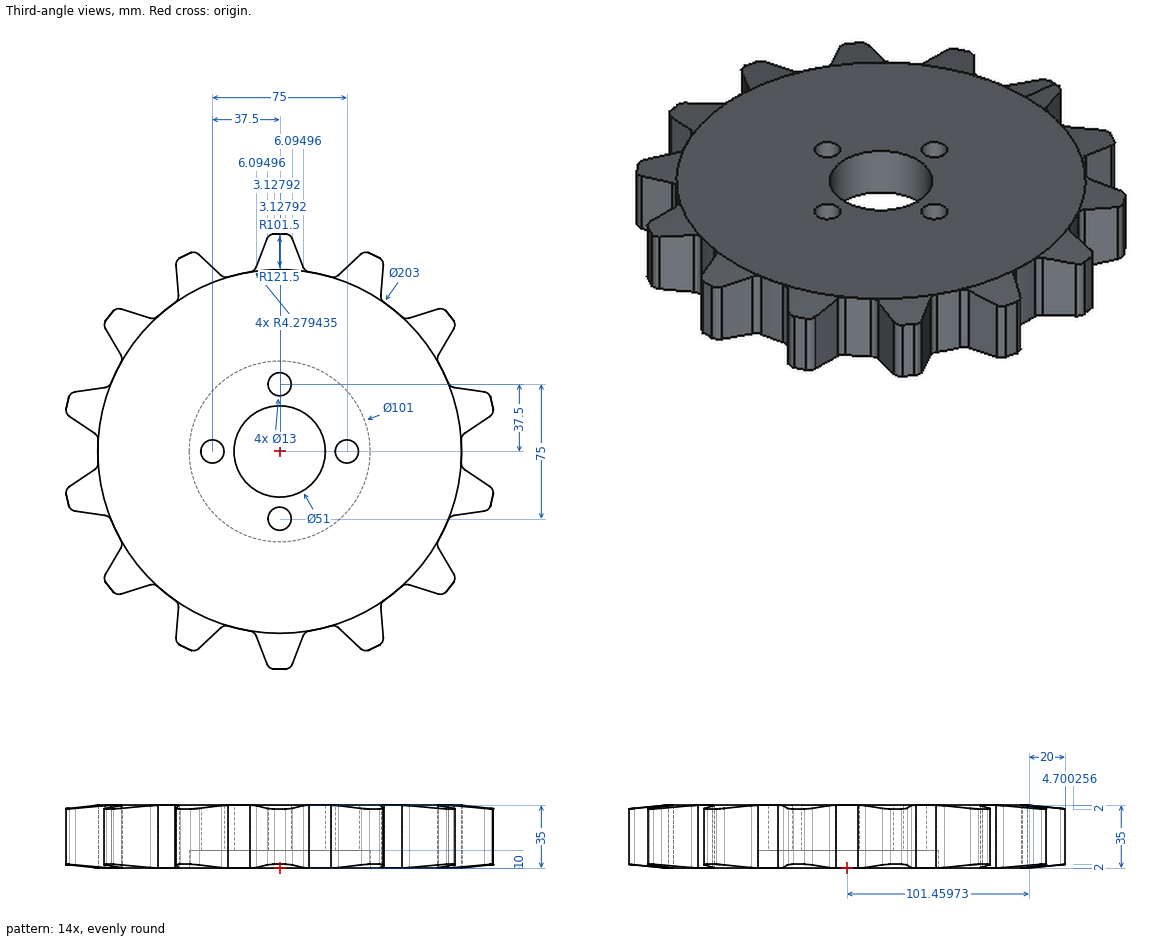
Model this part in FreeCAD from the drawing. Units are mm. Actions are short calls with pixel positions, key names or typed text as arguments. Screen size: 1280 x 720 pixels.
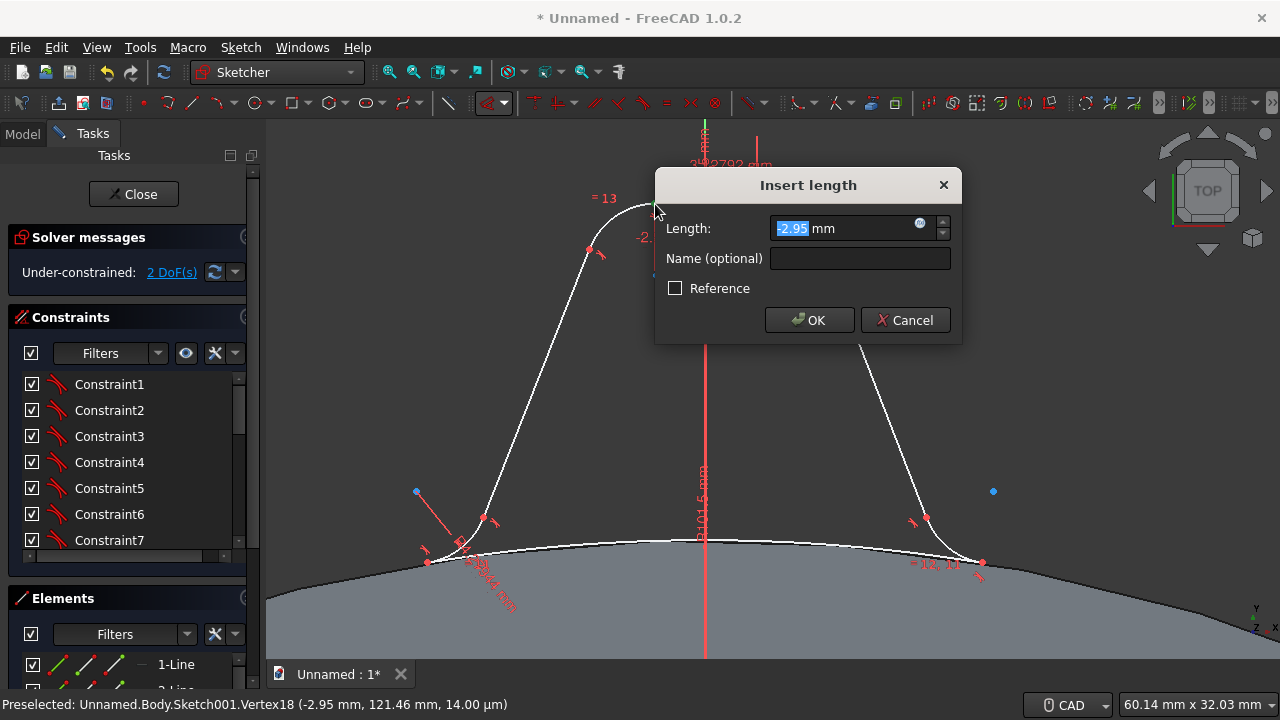
text(-3.12792)
key(Return)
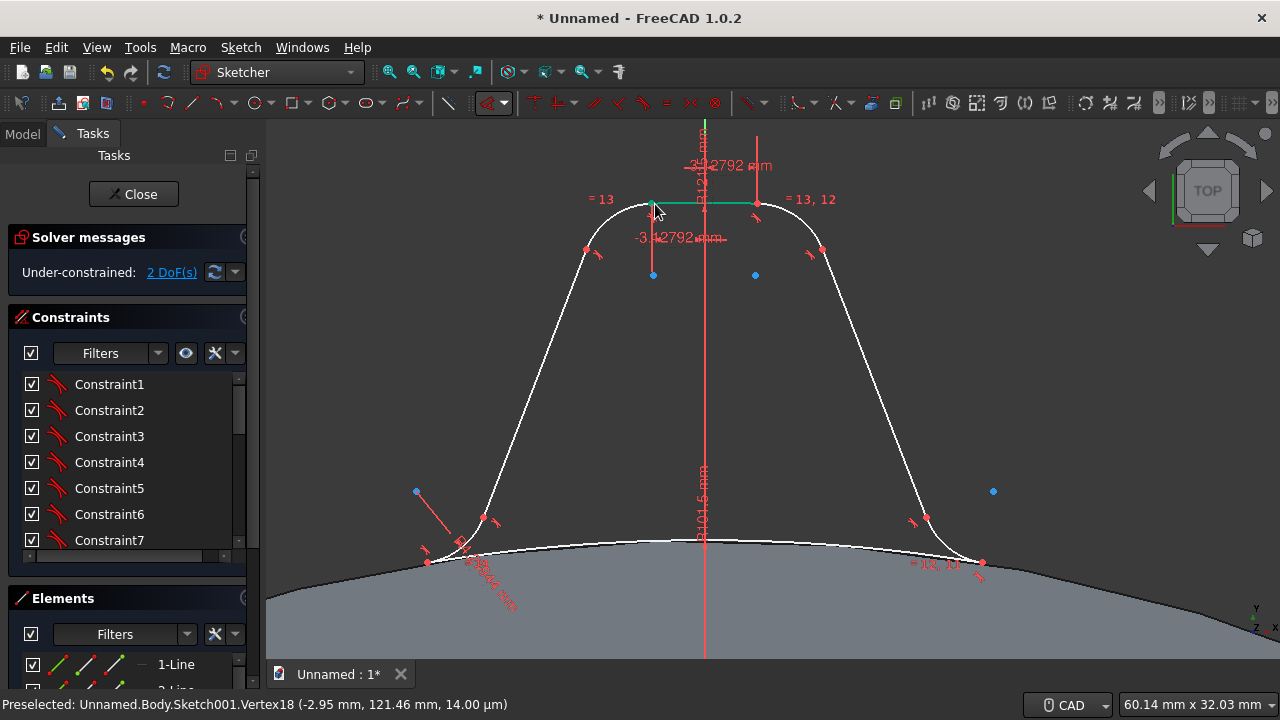
click(556, 330)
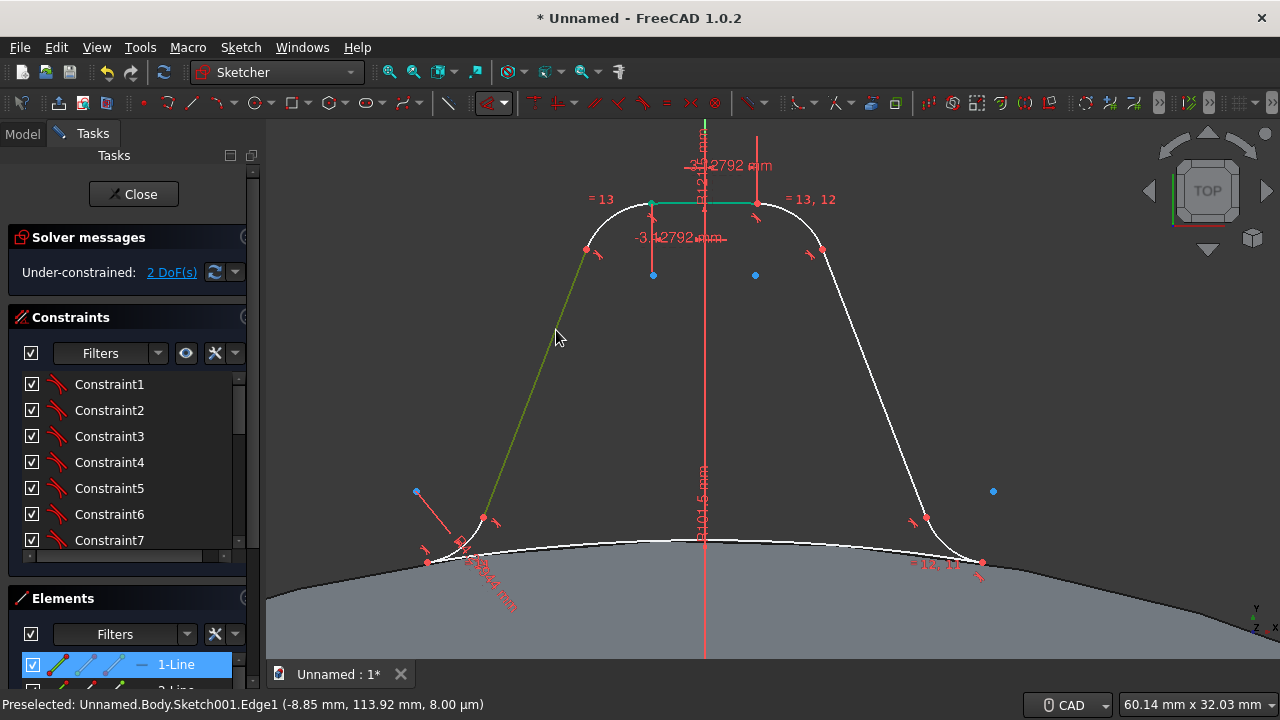
key(l)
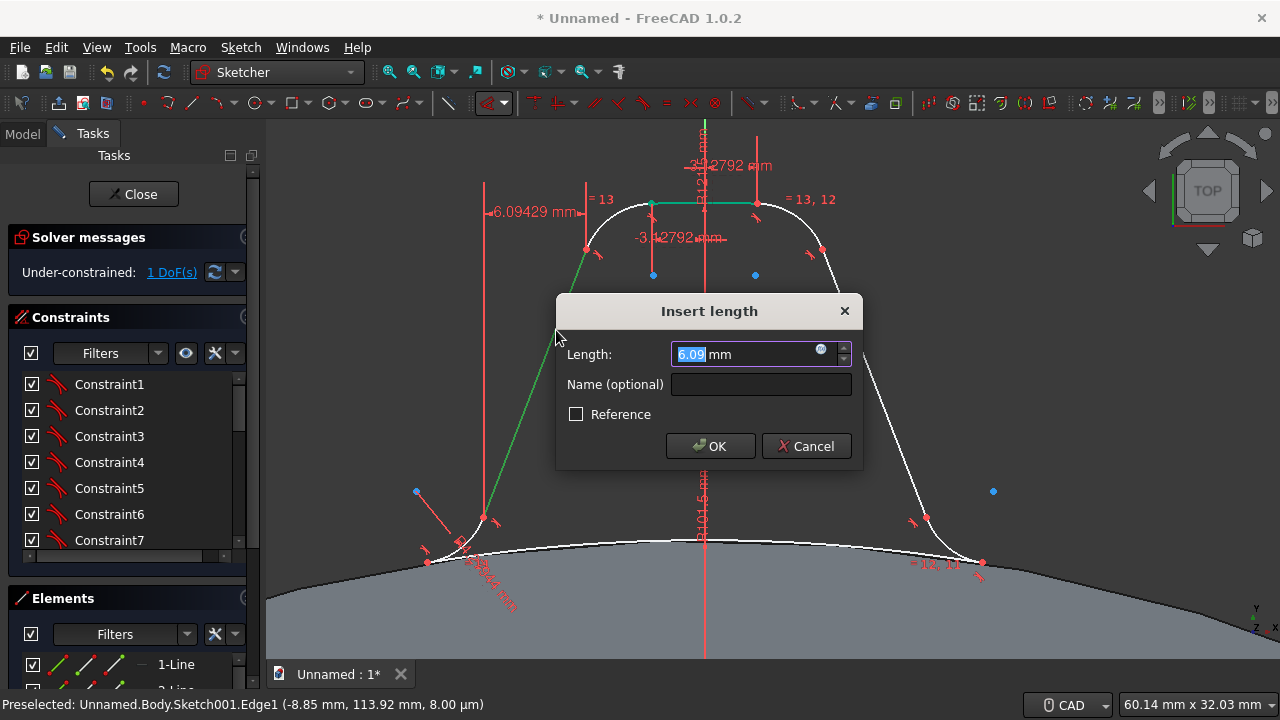
text(6.09496)
key(Return)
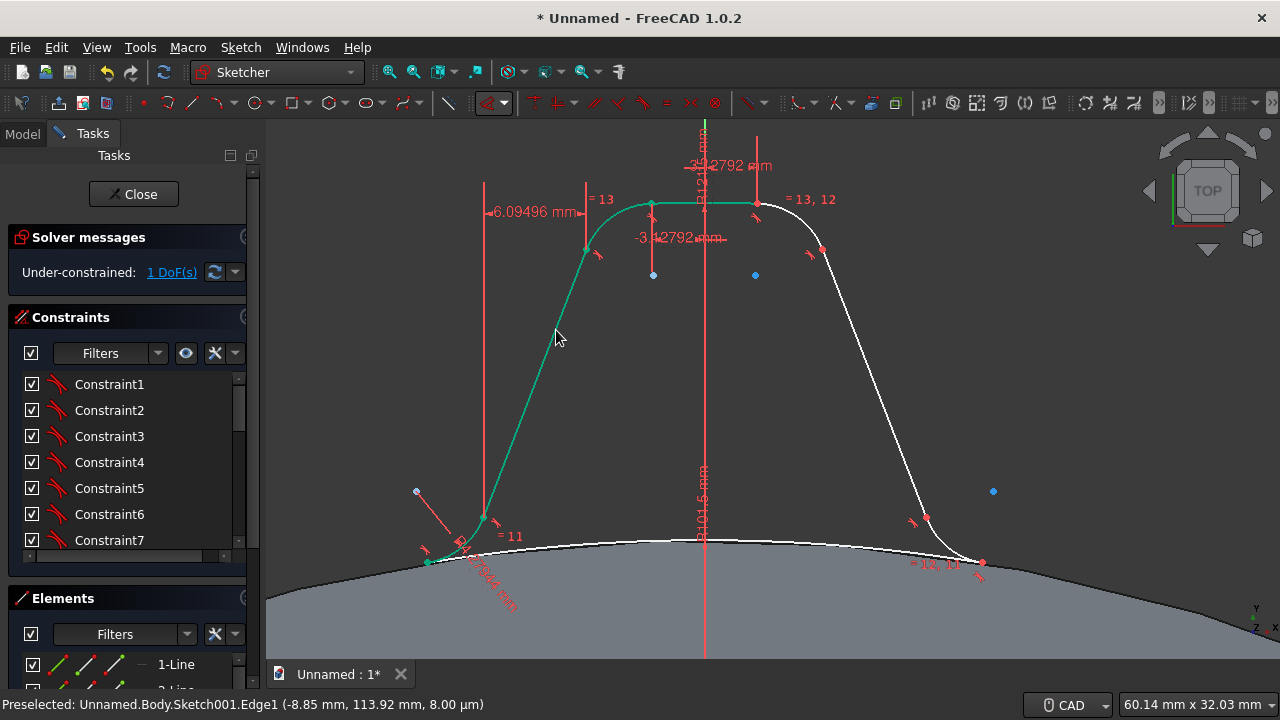
click(895, 437)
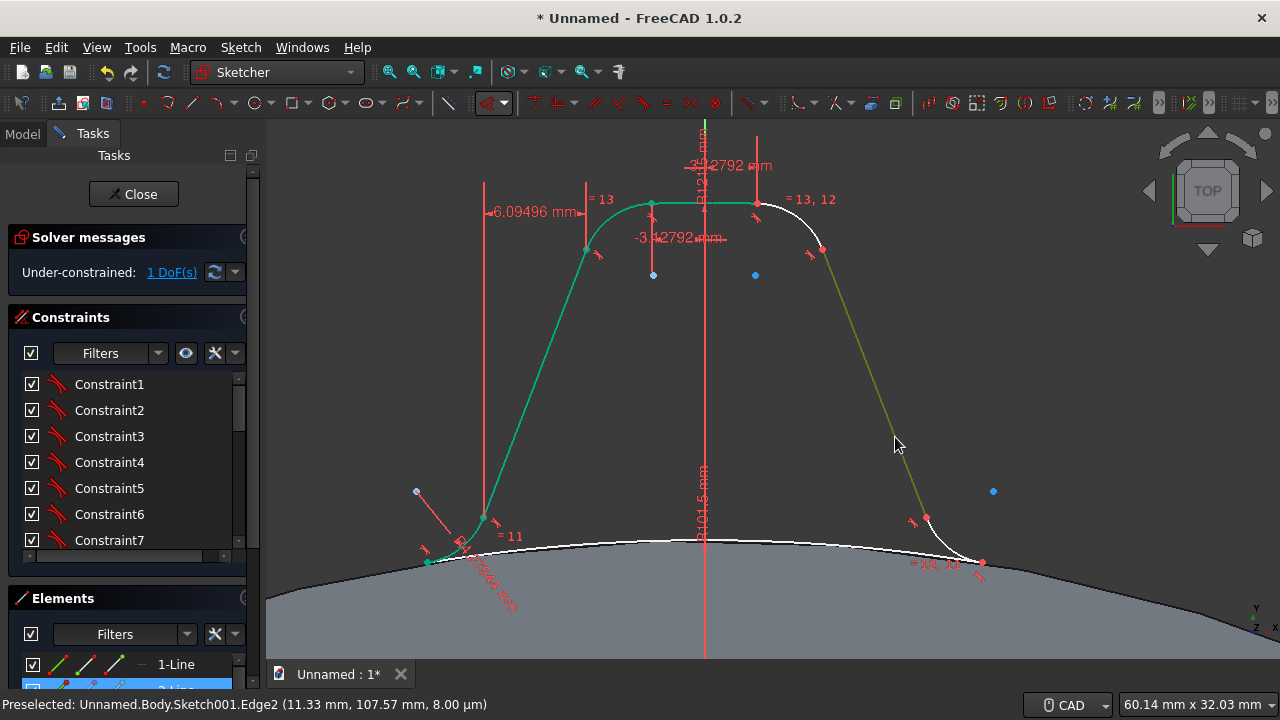
click(506, 104)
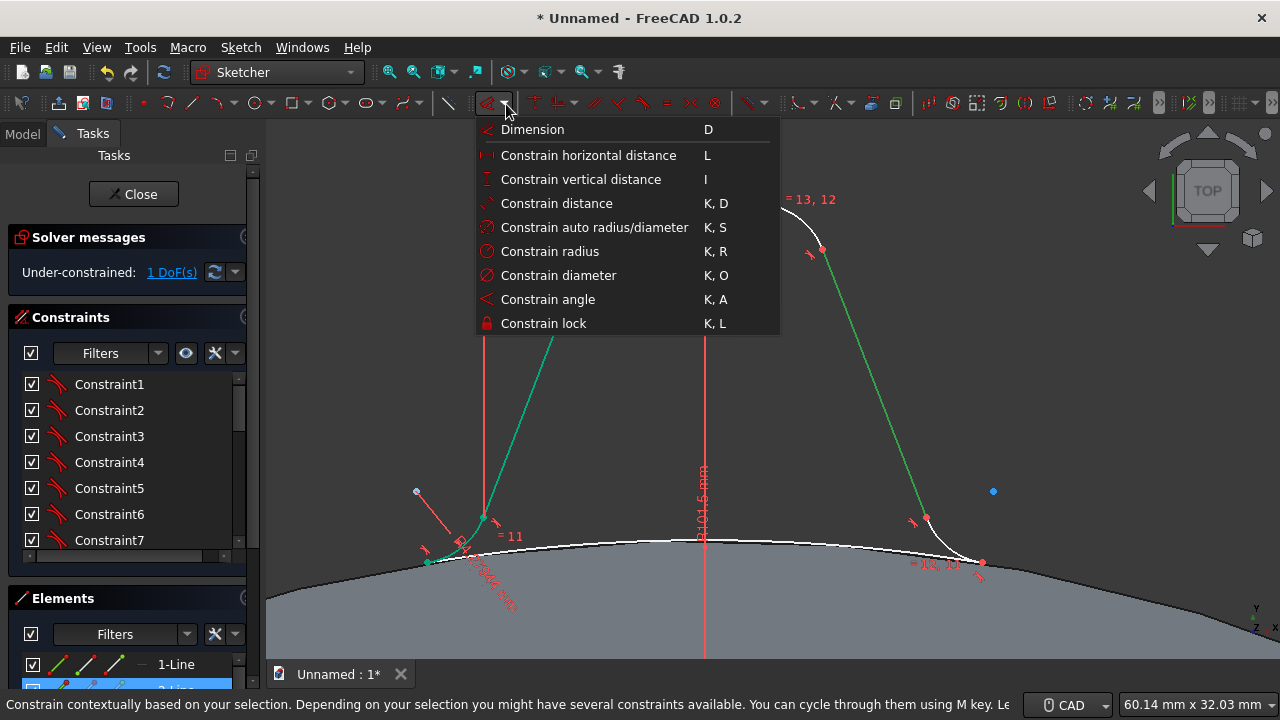
click(628, 155)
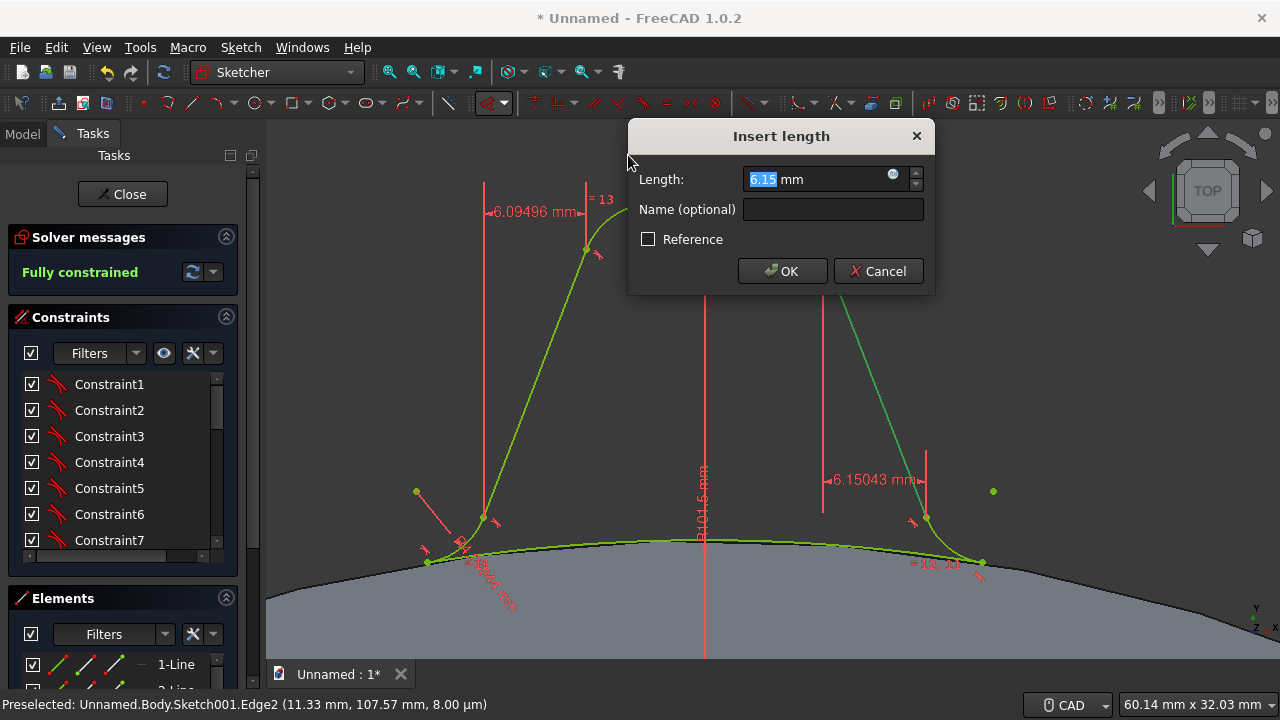
text(6.09496)
key(Return)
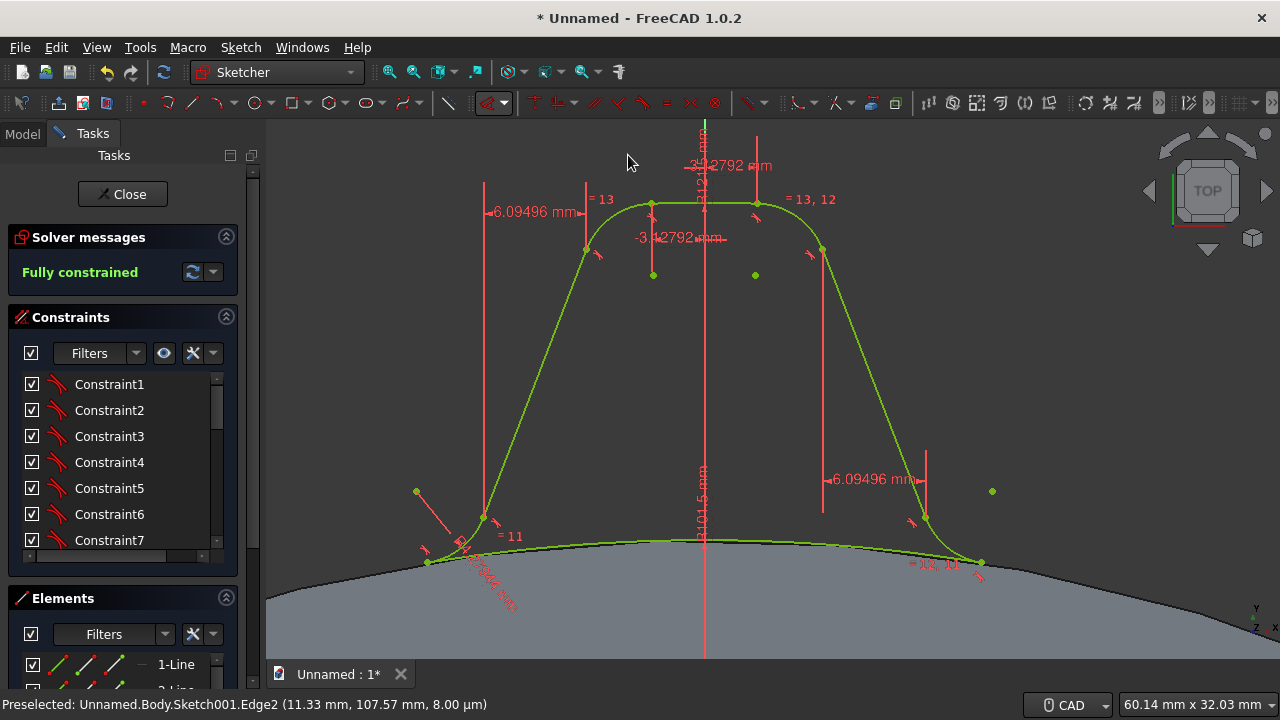
click(123, 194)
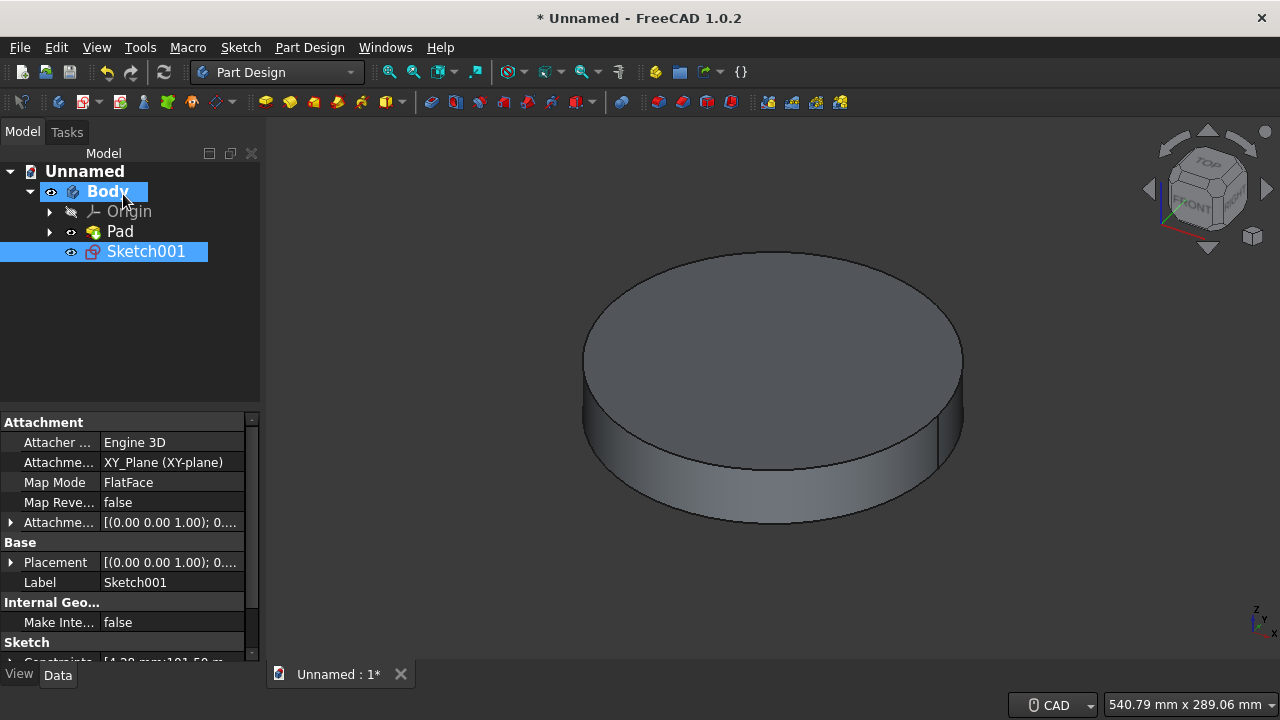
click(266, 102)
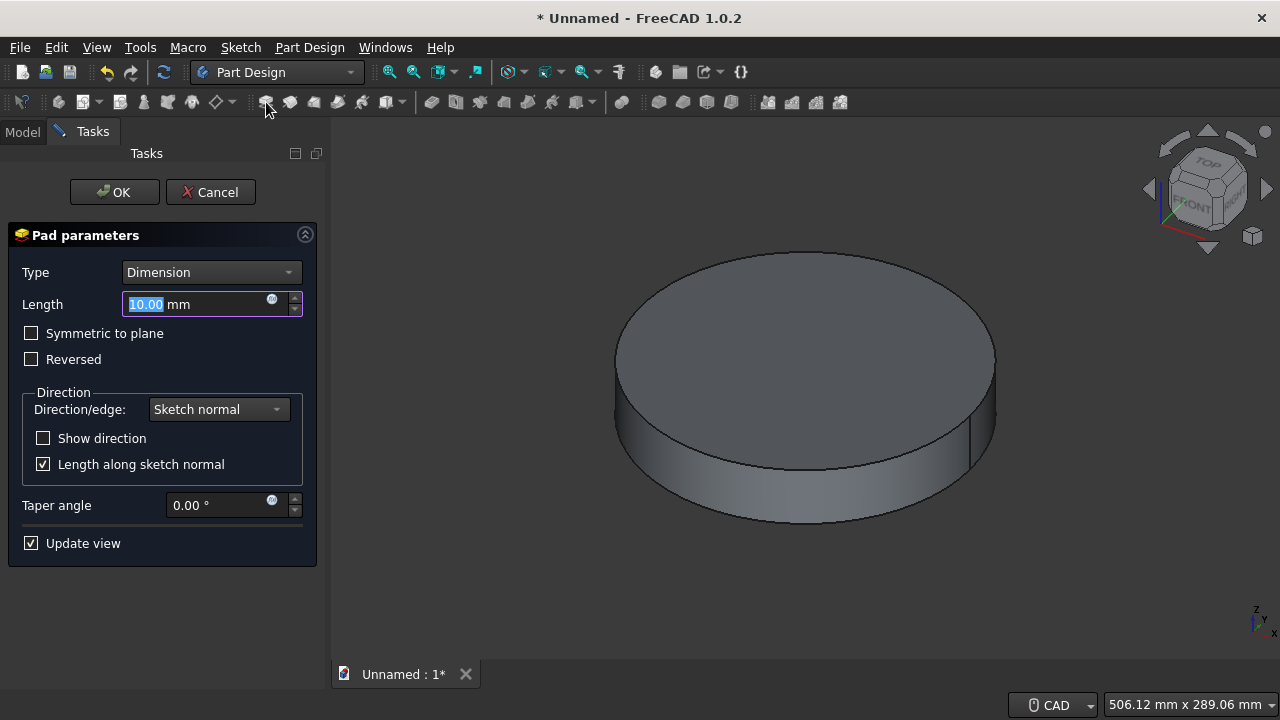
text(35)
key(Tab)